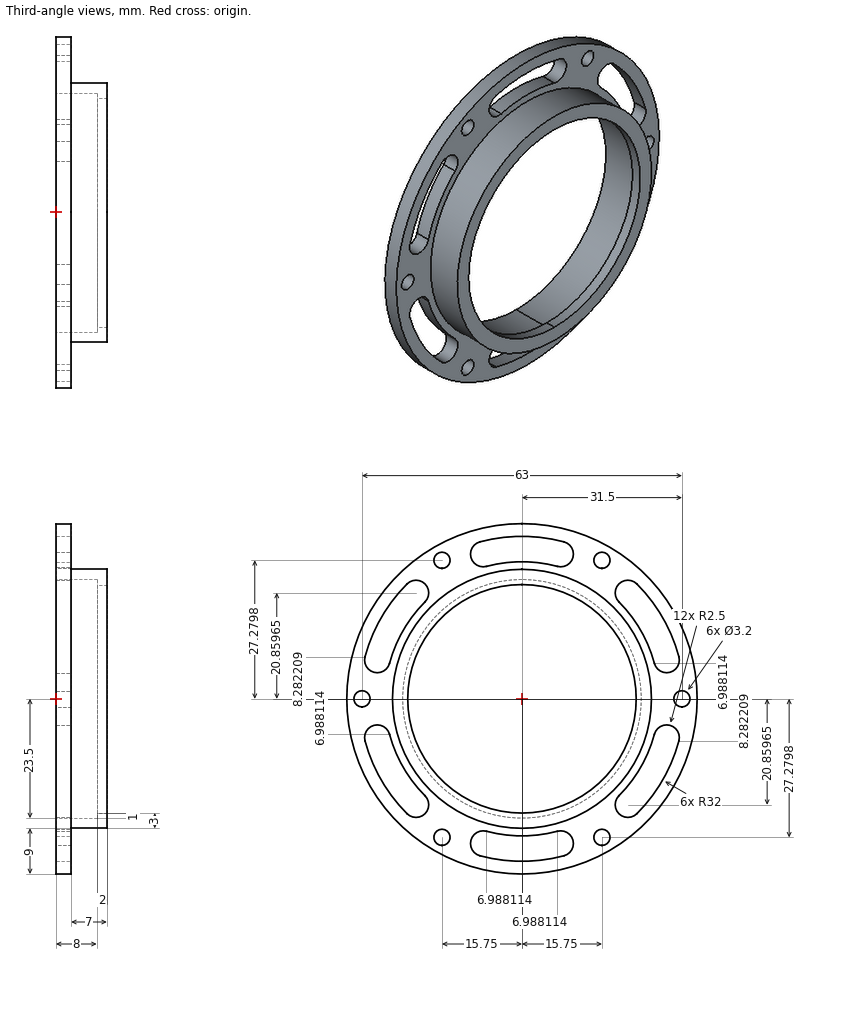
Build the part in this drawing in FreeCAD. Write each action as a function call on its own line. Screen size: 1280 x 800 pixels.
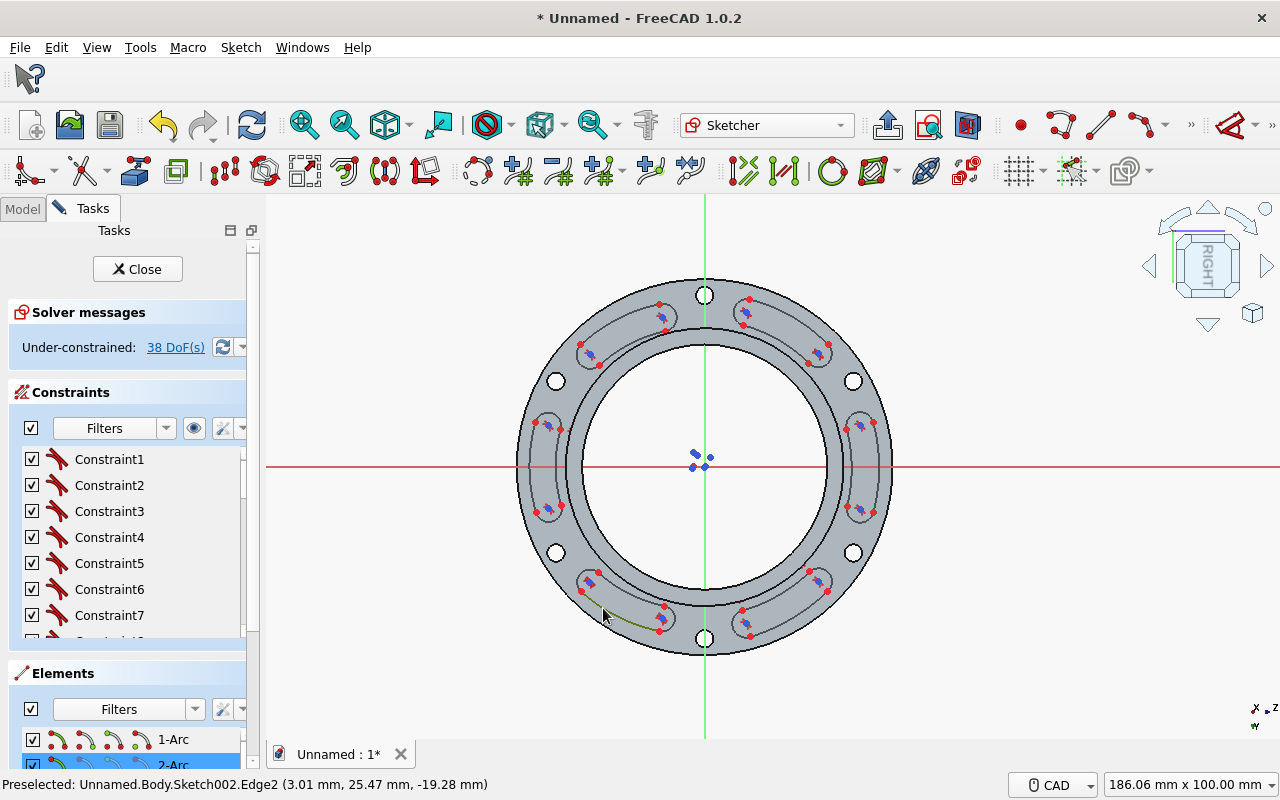
click(807, 327)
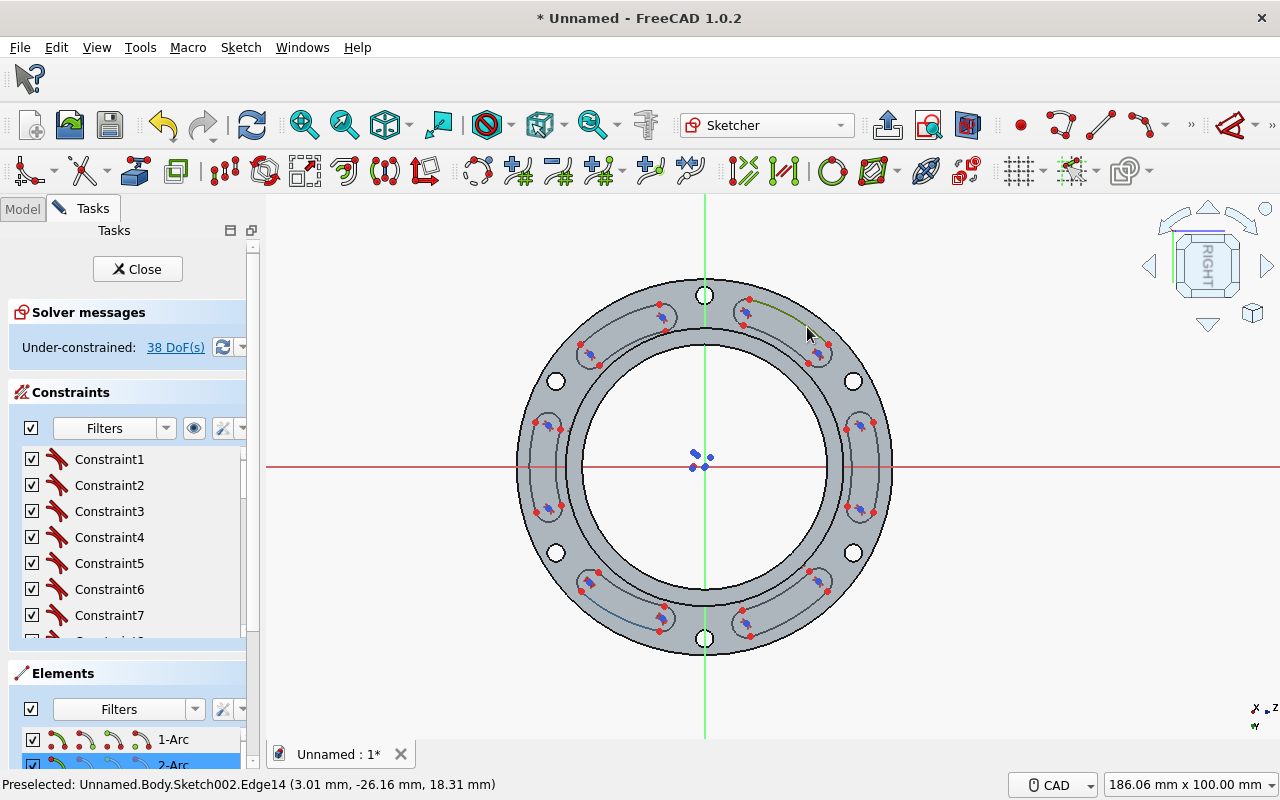
key(c)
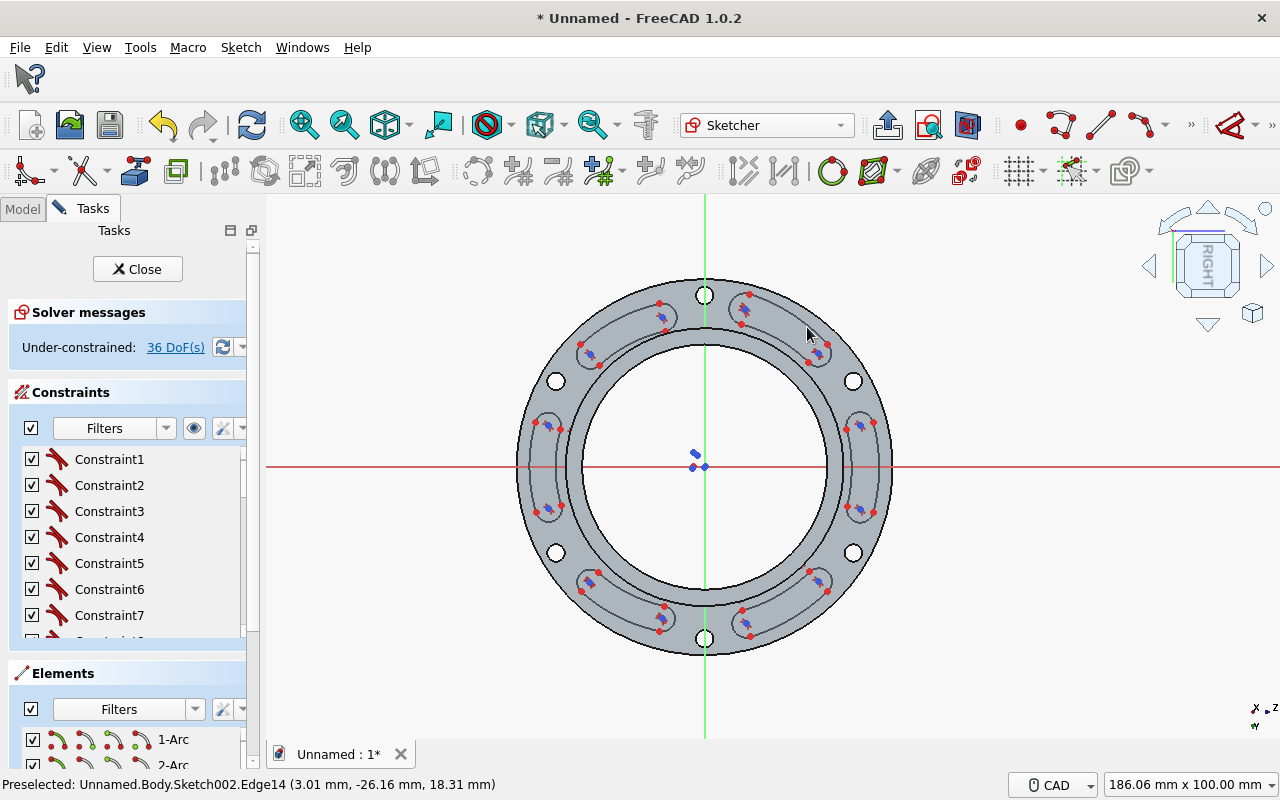
click(603, 608)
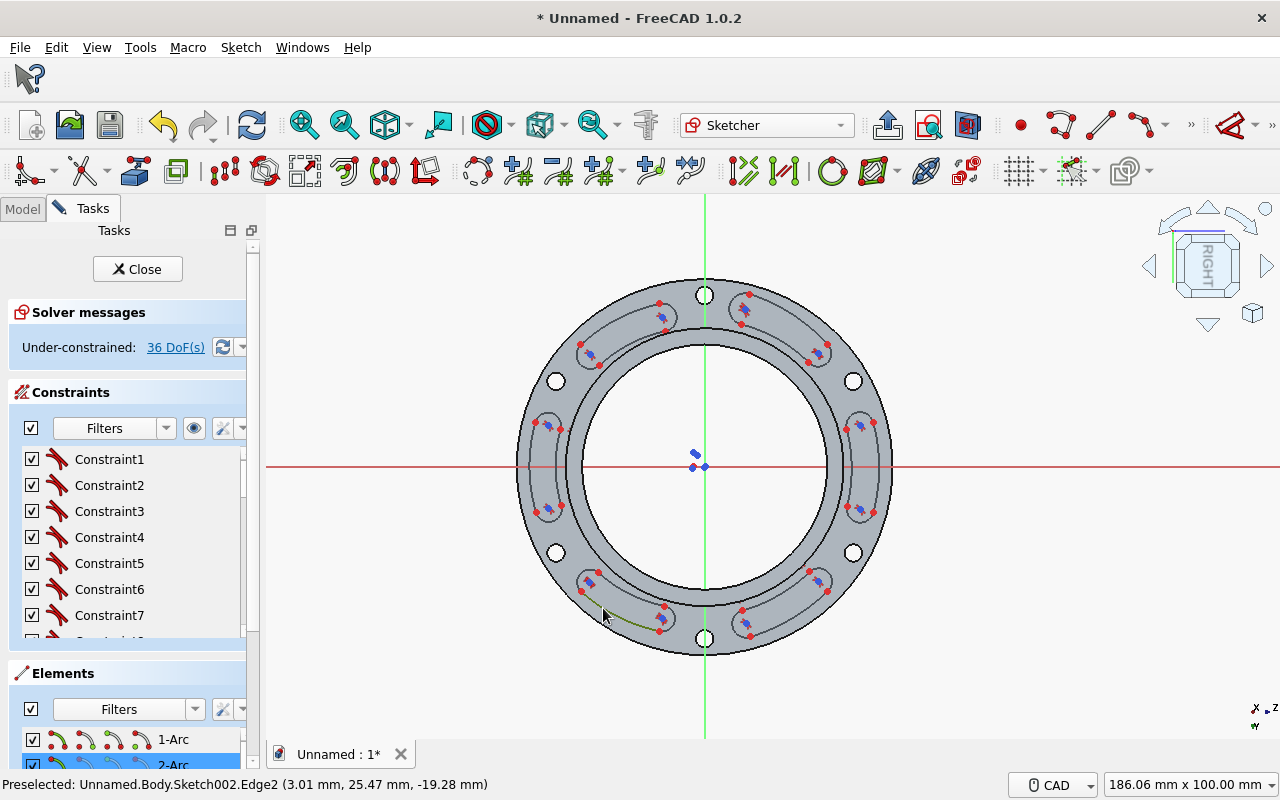
click(791, 347)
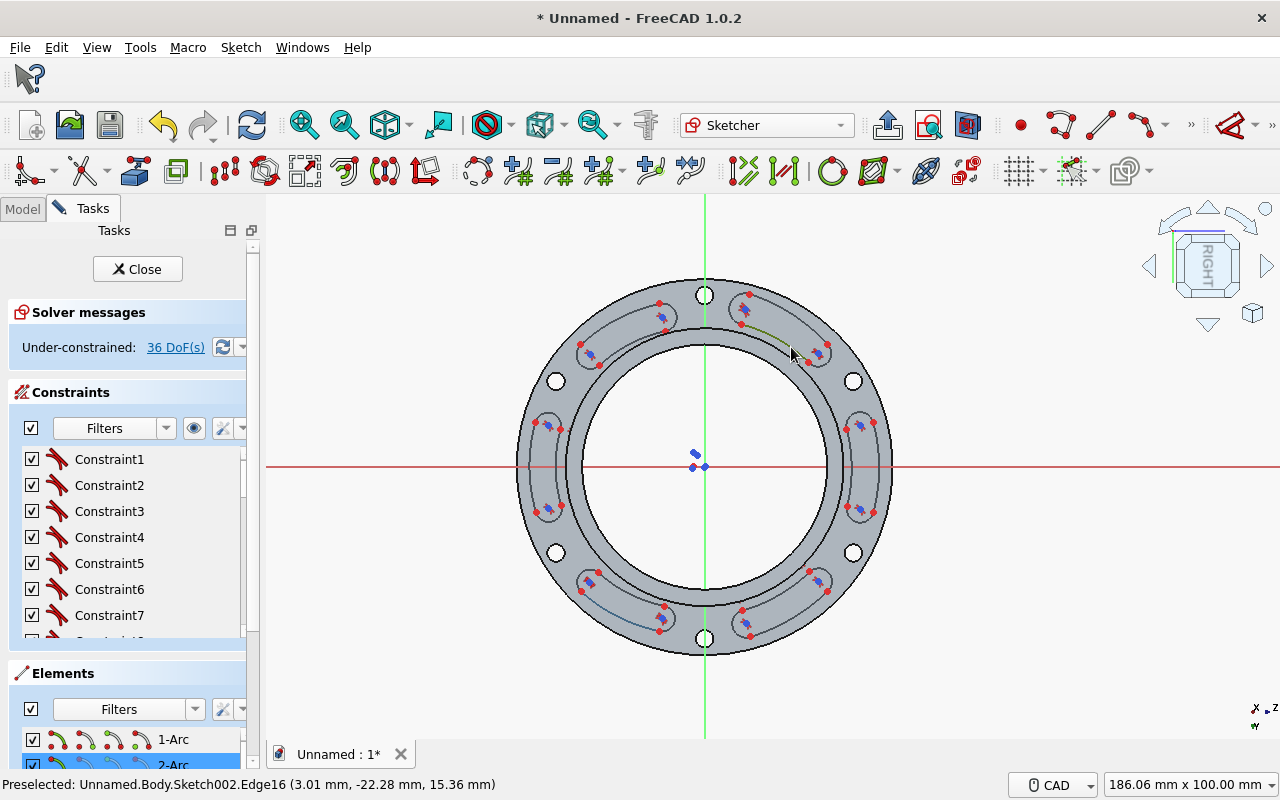
key(c)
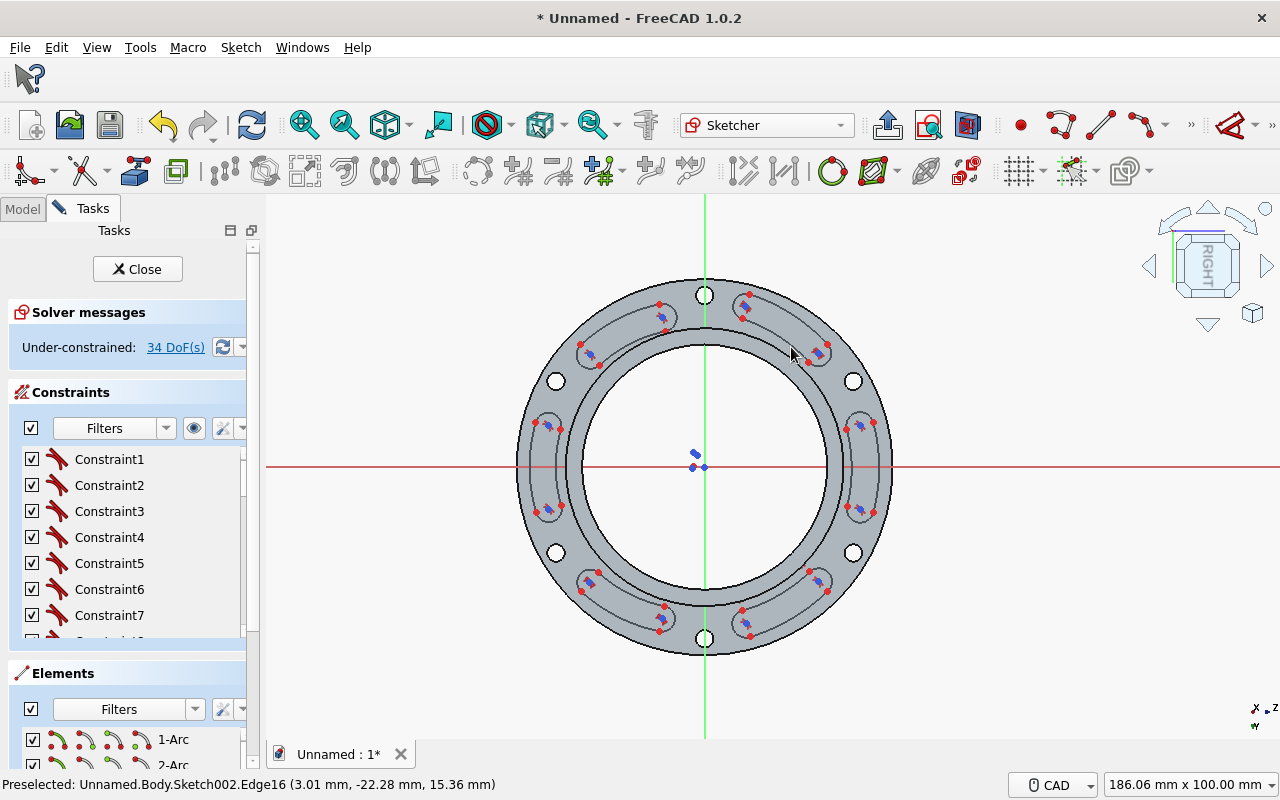
click(603, 608)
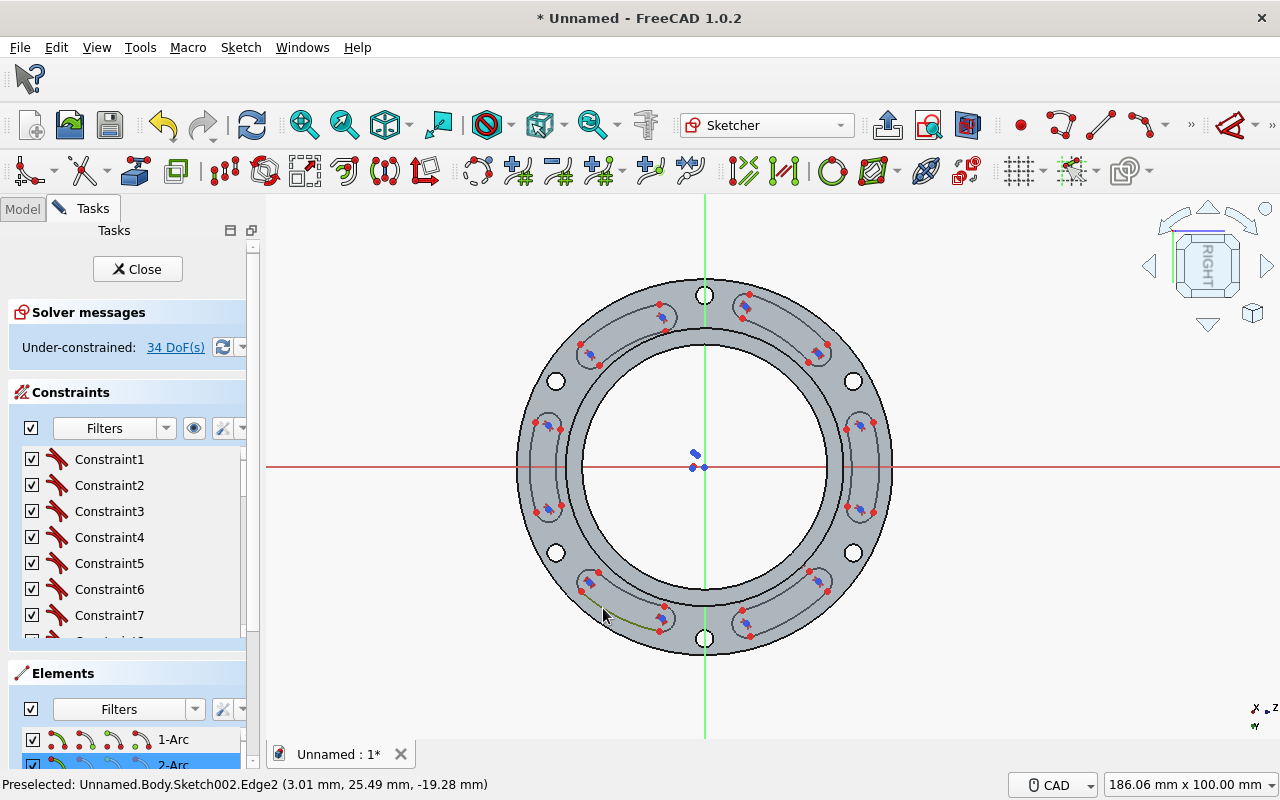
click(851, 483)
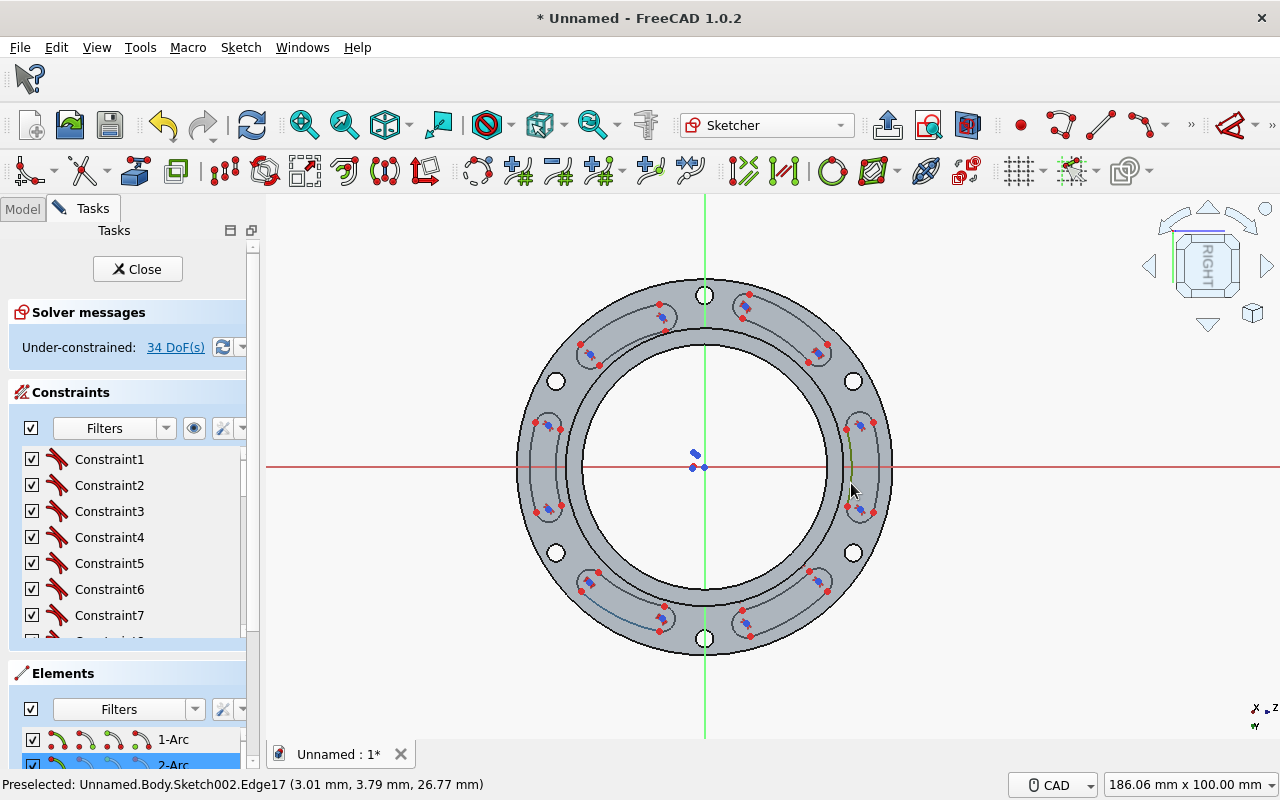
key(c)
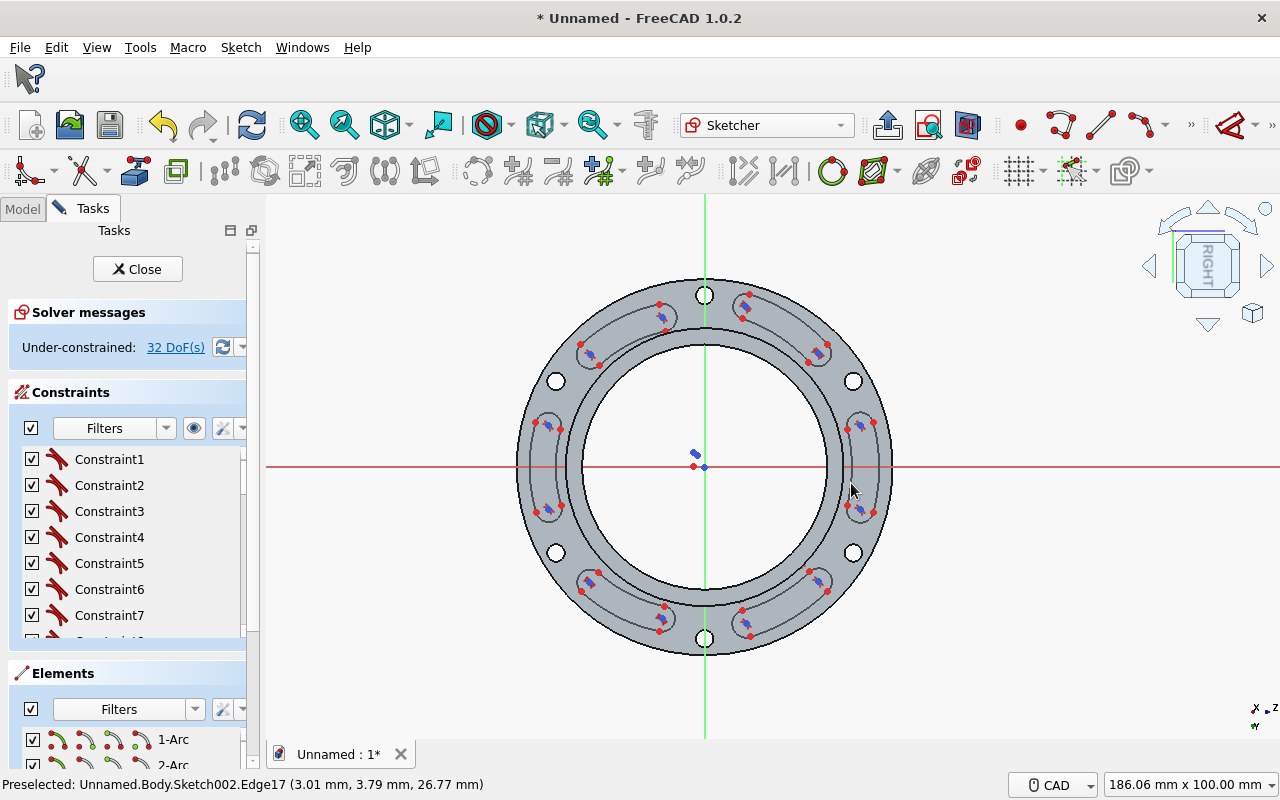
click(603, 608)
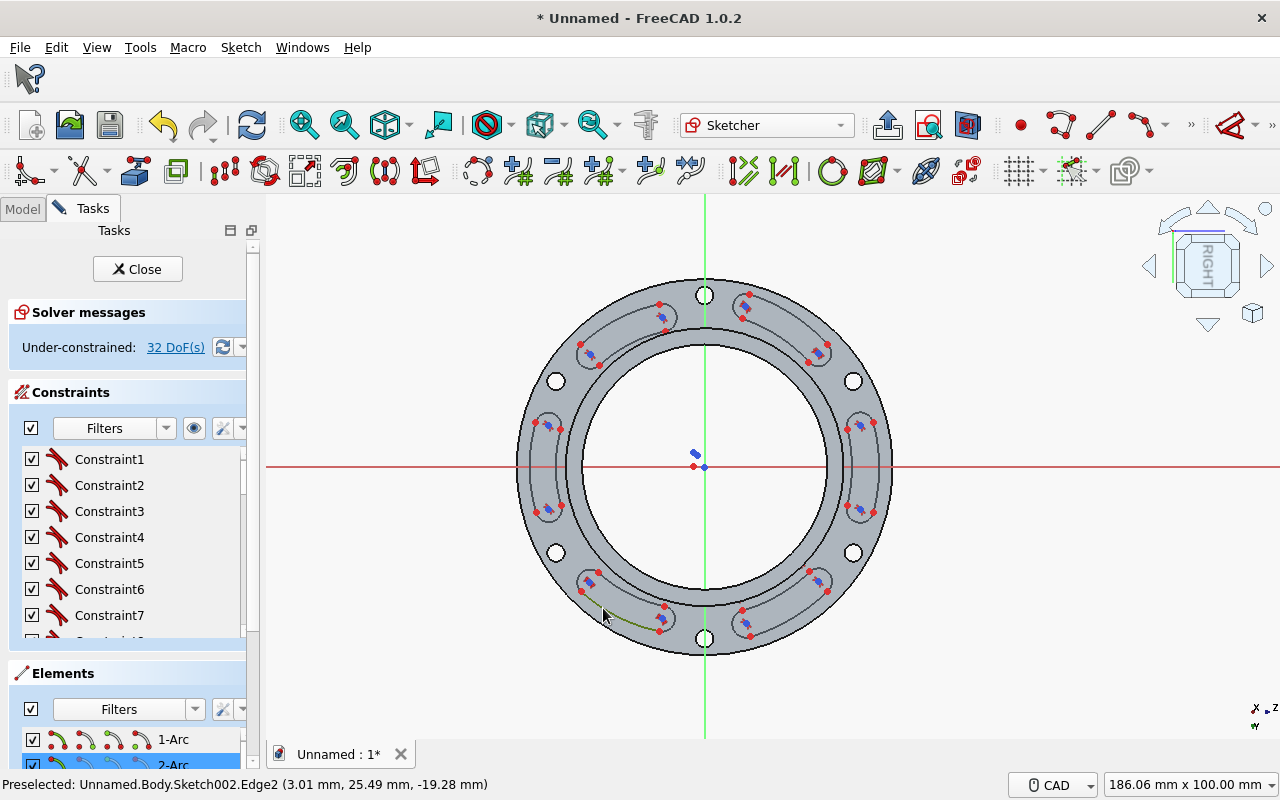
click(878, 486)